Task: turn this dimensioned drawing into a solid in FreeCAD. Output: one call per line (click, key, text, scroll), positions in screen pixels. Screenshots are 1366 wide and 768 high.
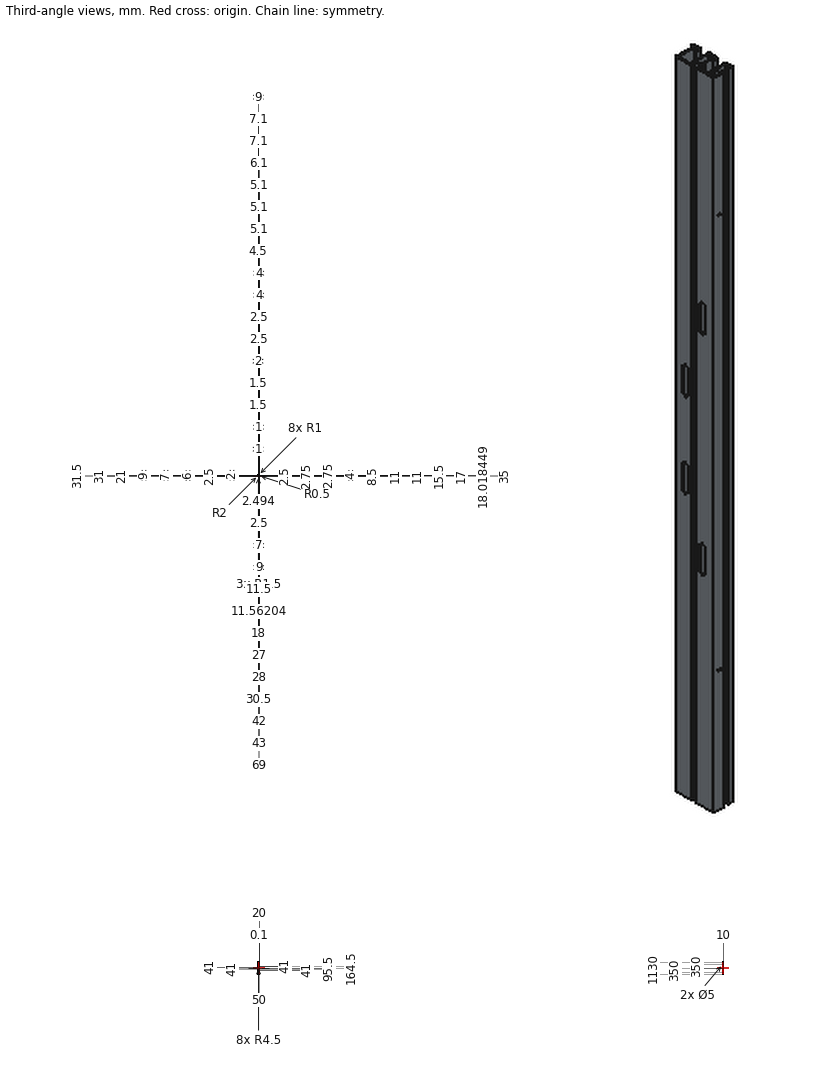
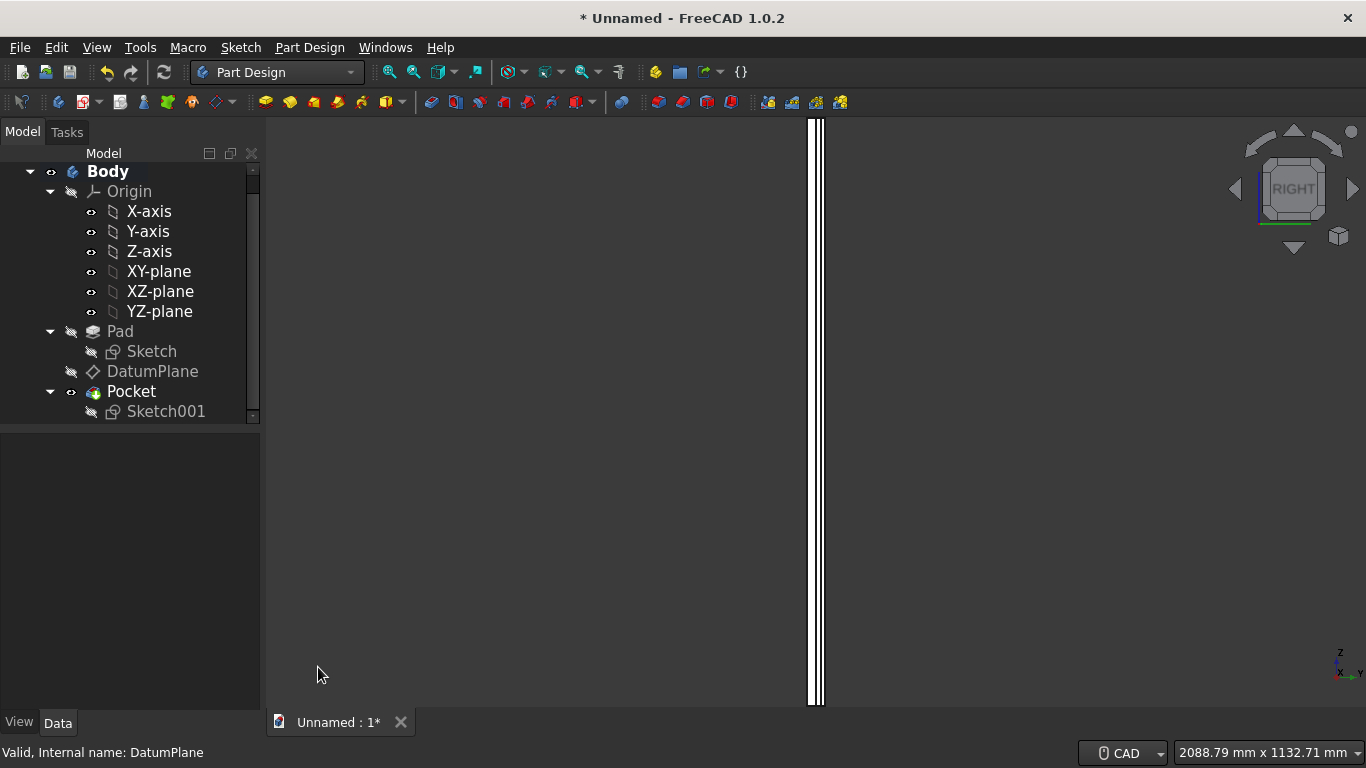
click(84, 102)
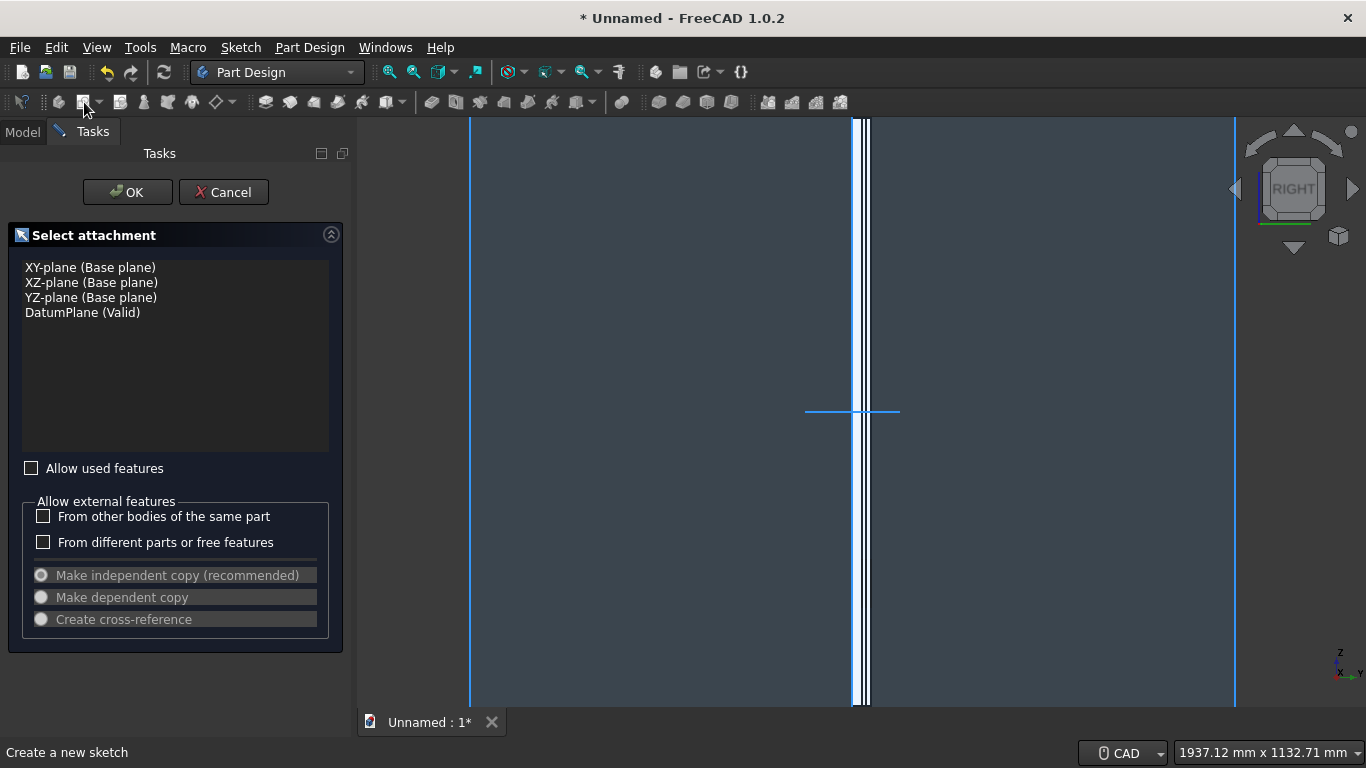
click(82, 298)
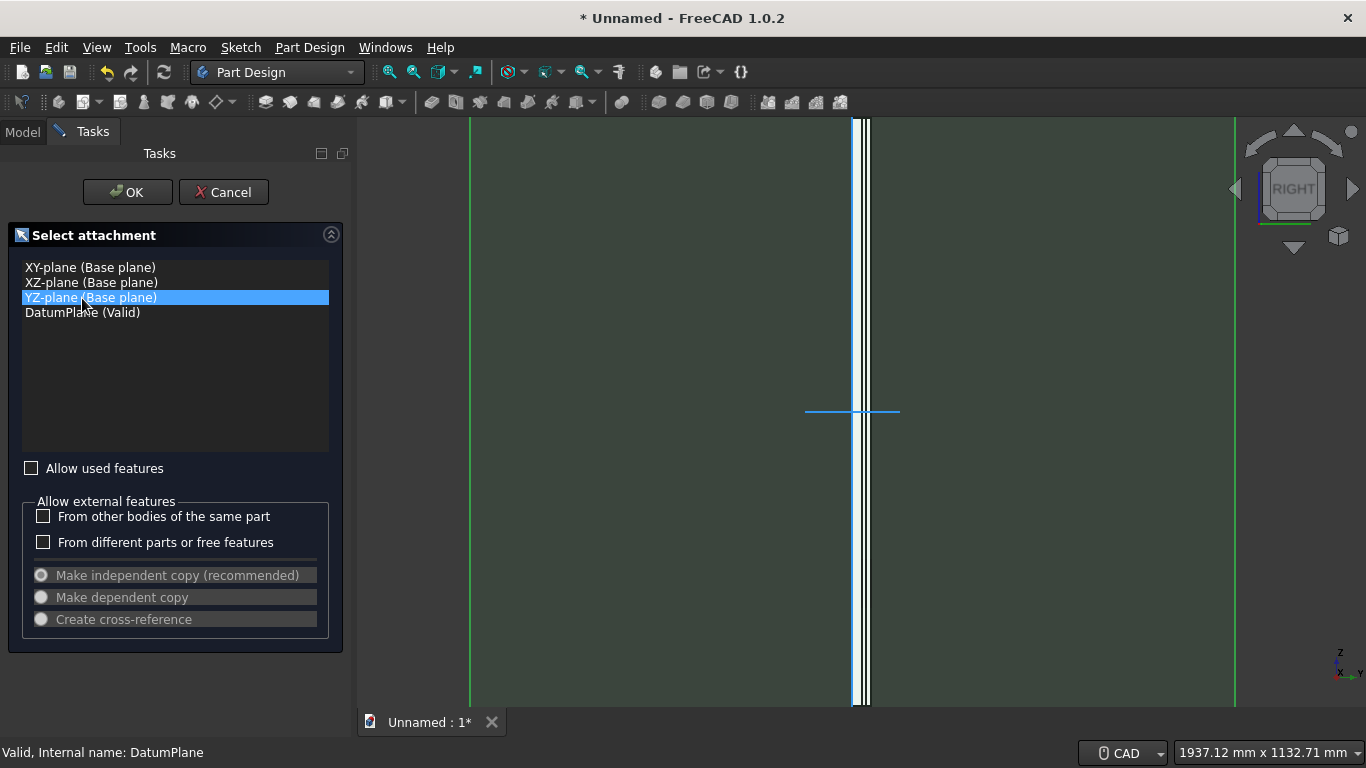
click(128, 192)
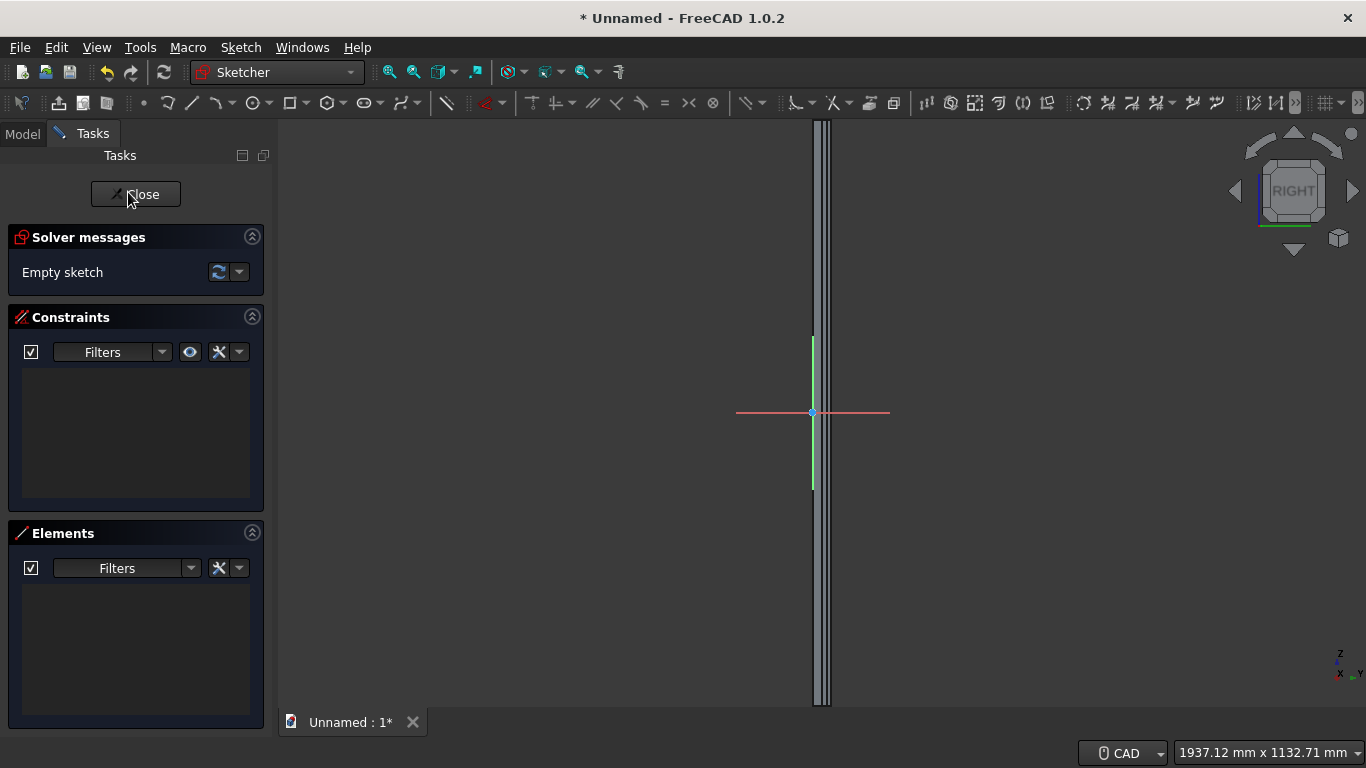
click(254, 104)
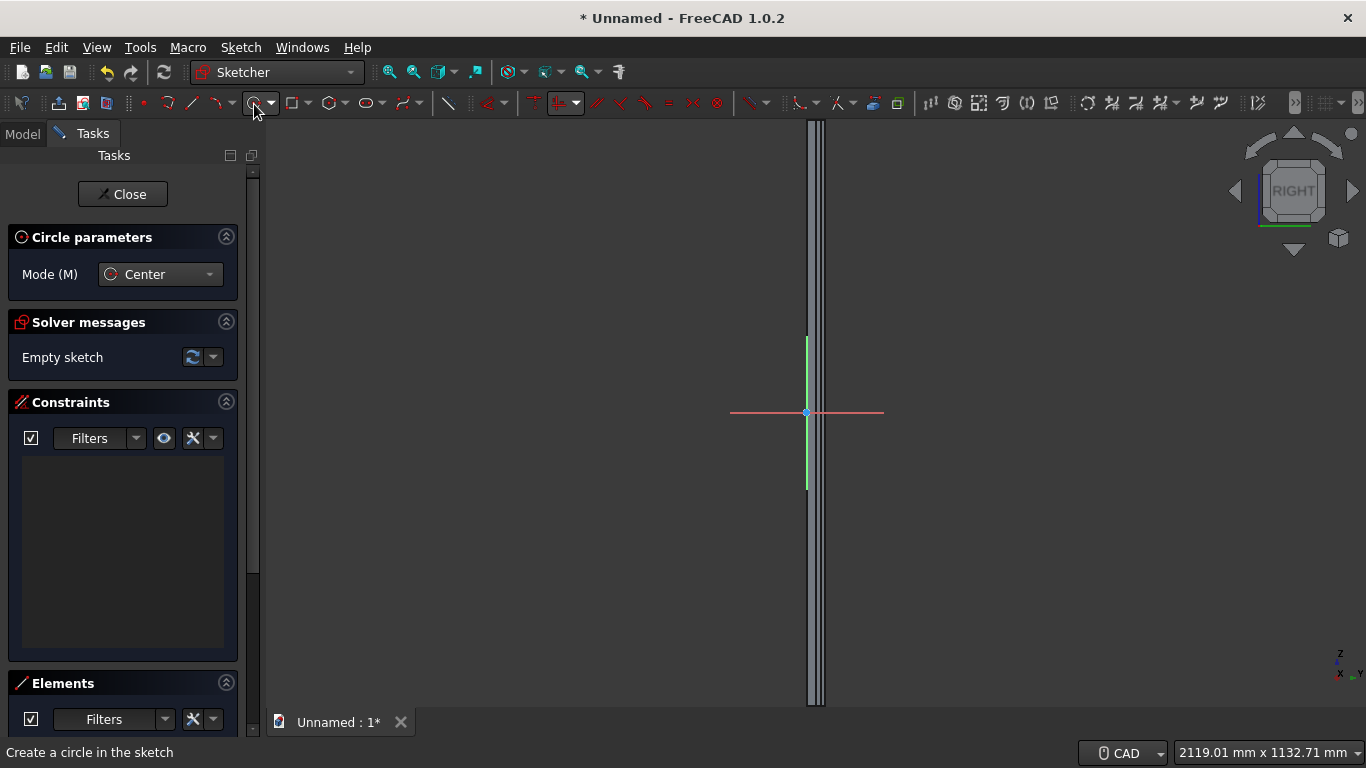
scroll(812, 231, up, 15)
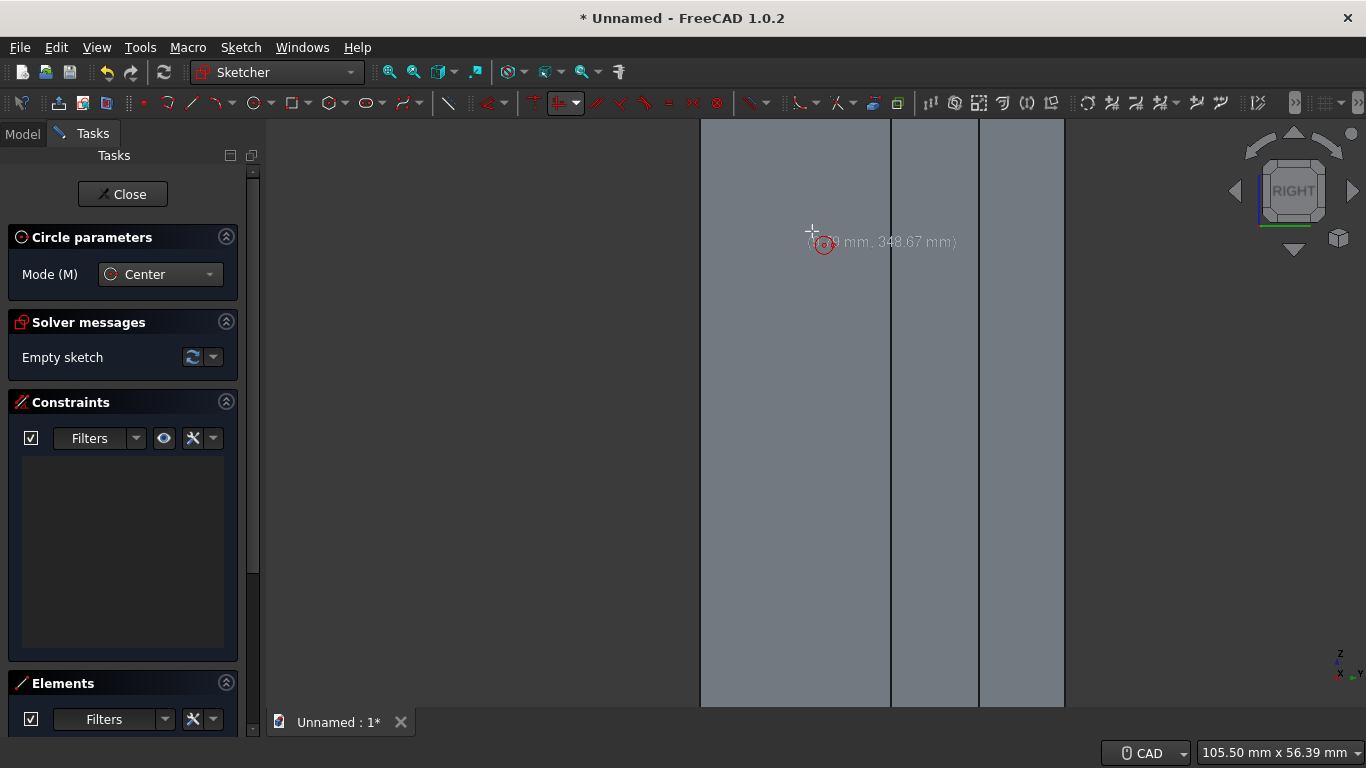
scroll(747, 231, down, 15)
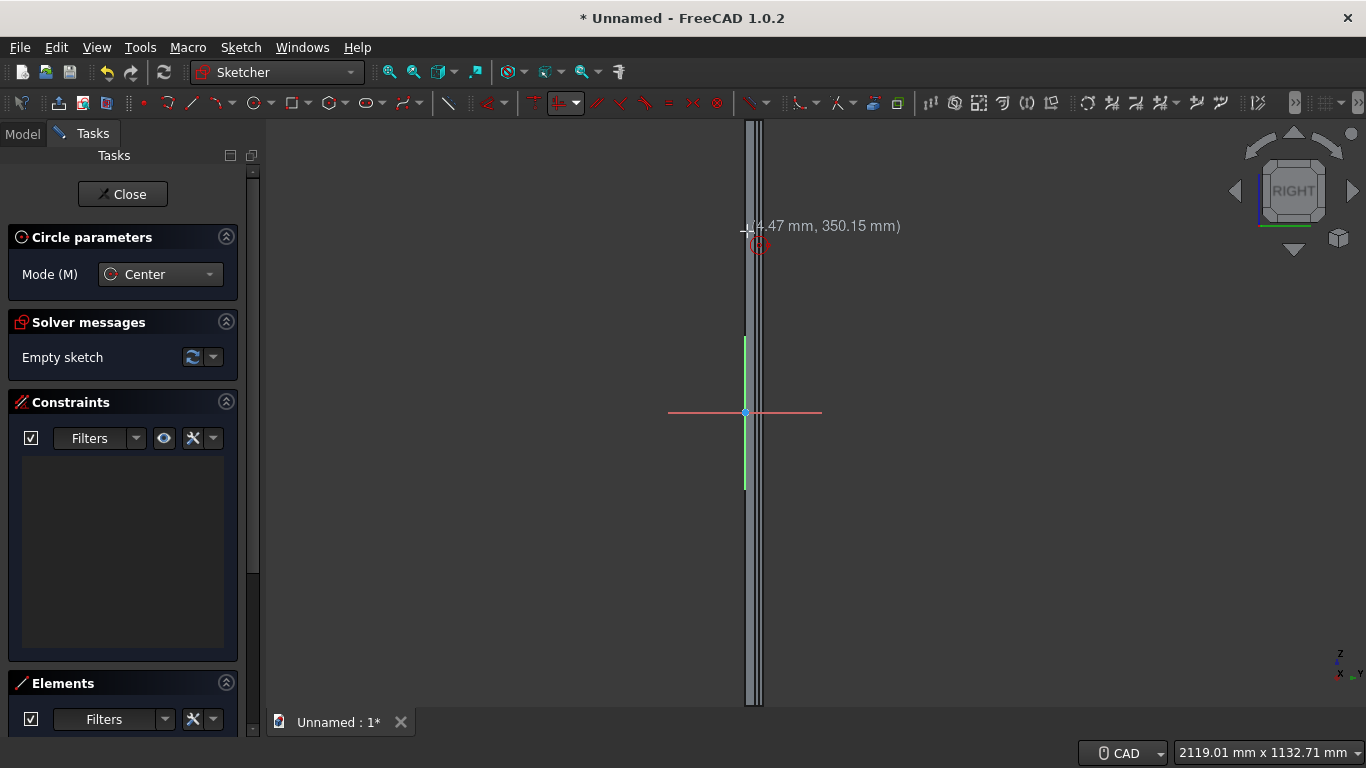
scroll(750, 231, up, 6)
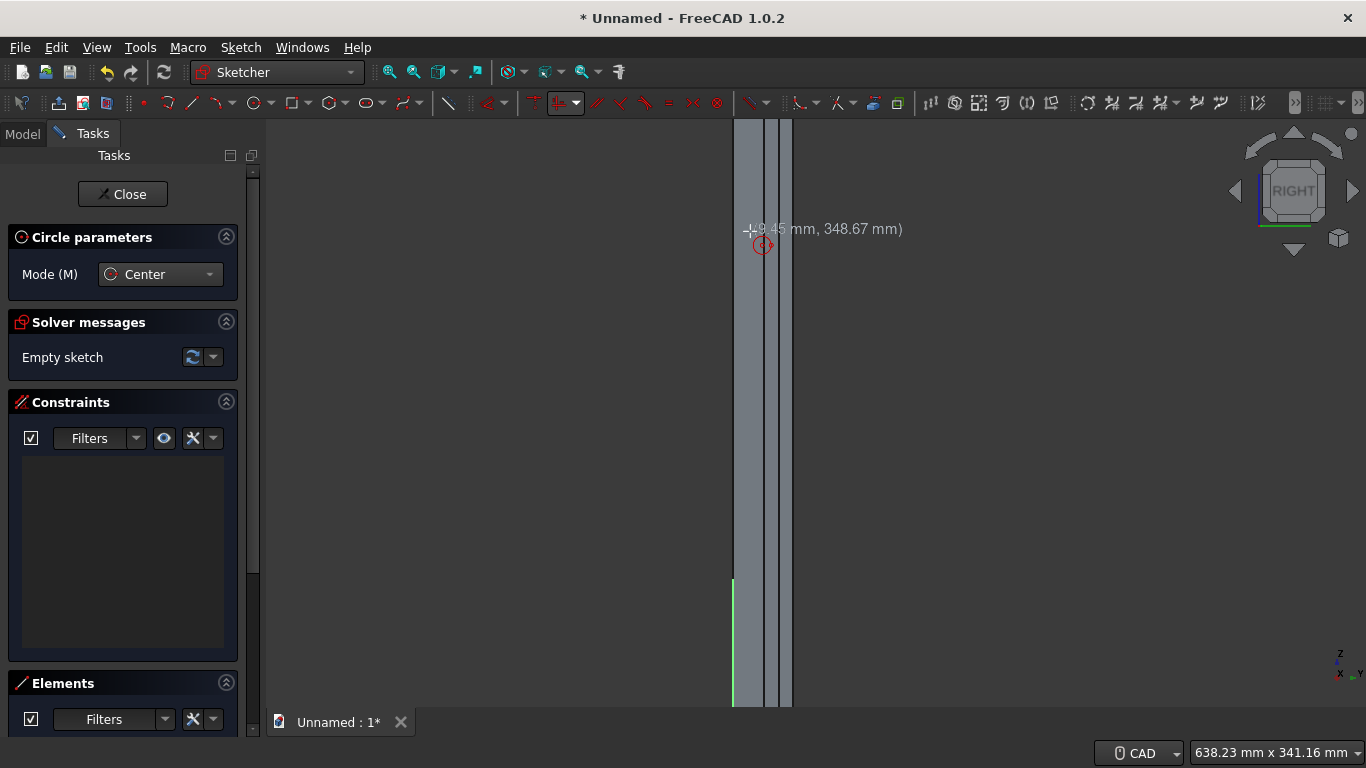
click(750, 232)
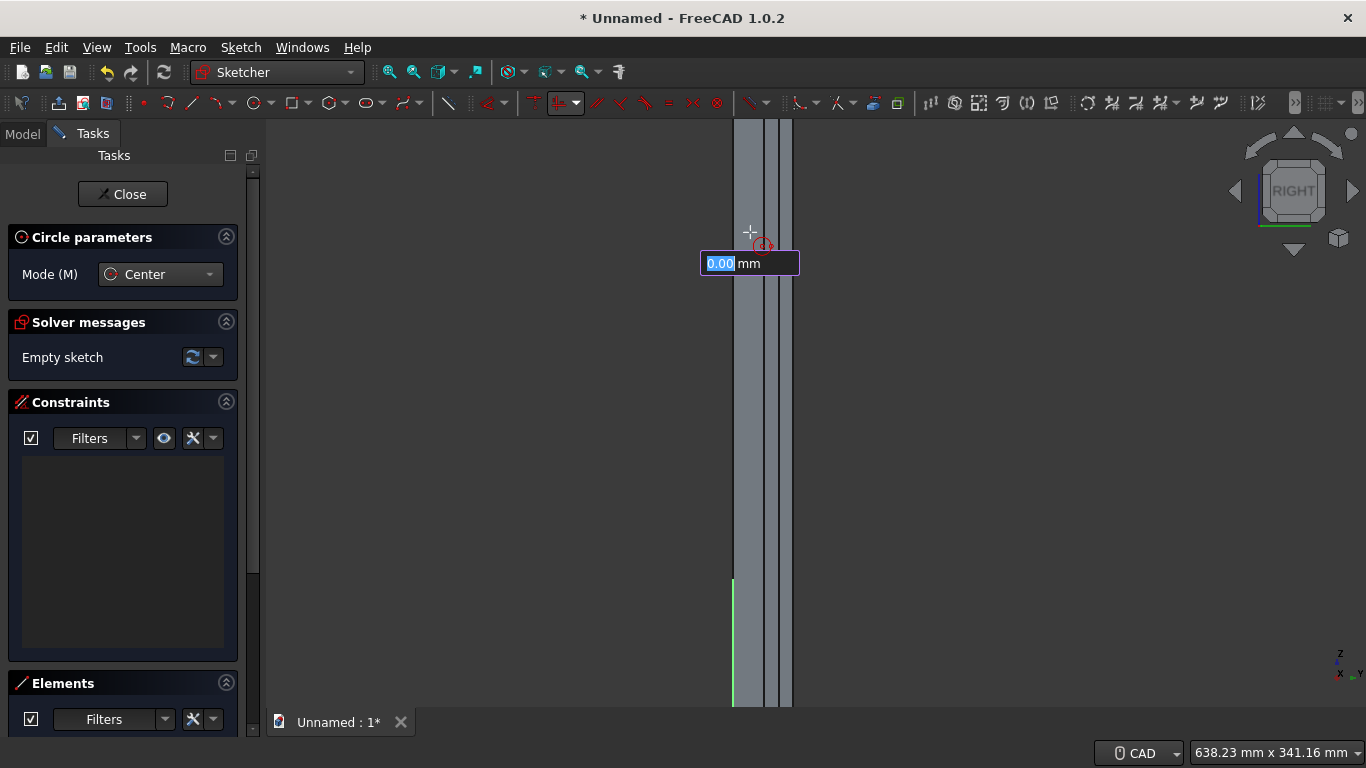
scroll(753, 229, up, 7)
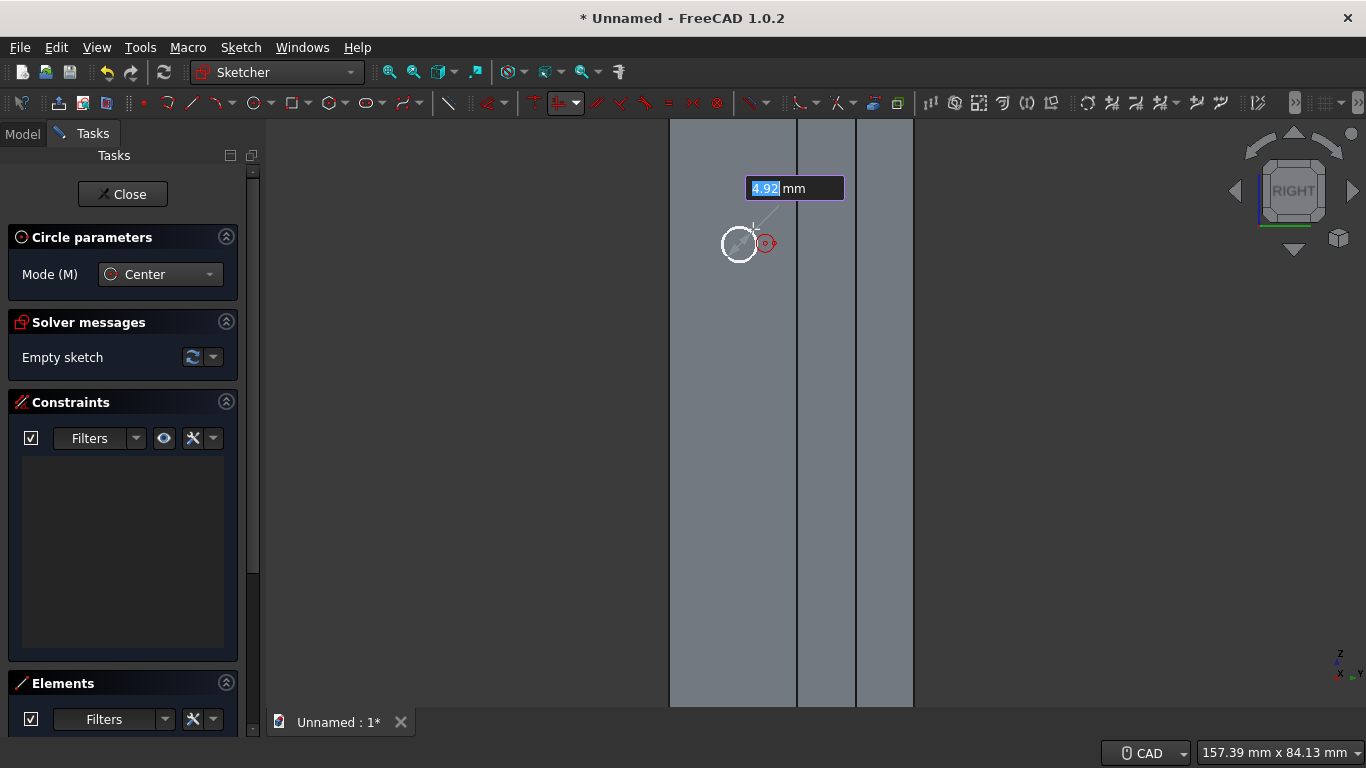
click(752, 227)